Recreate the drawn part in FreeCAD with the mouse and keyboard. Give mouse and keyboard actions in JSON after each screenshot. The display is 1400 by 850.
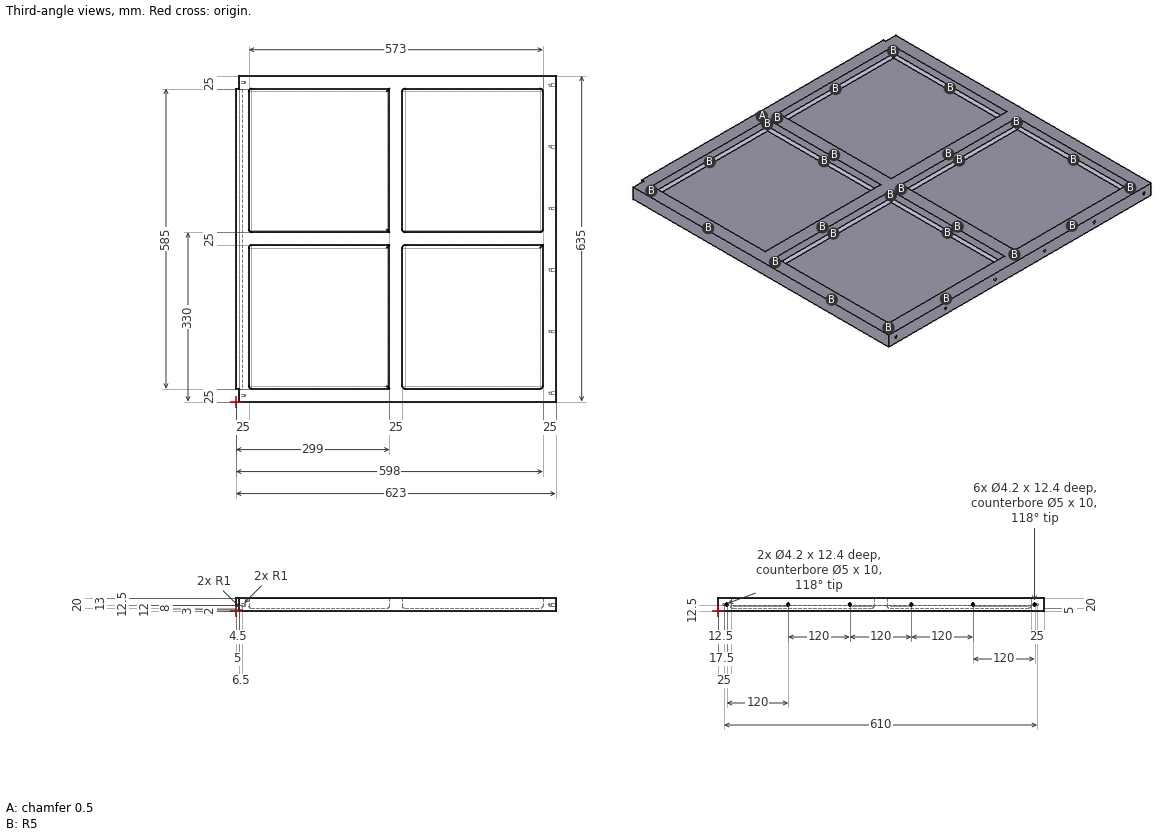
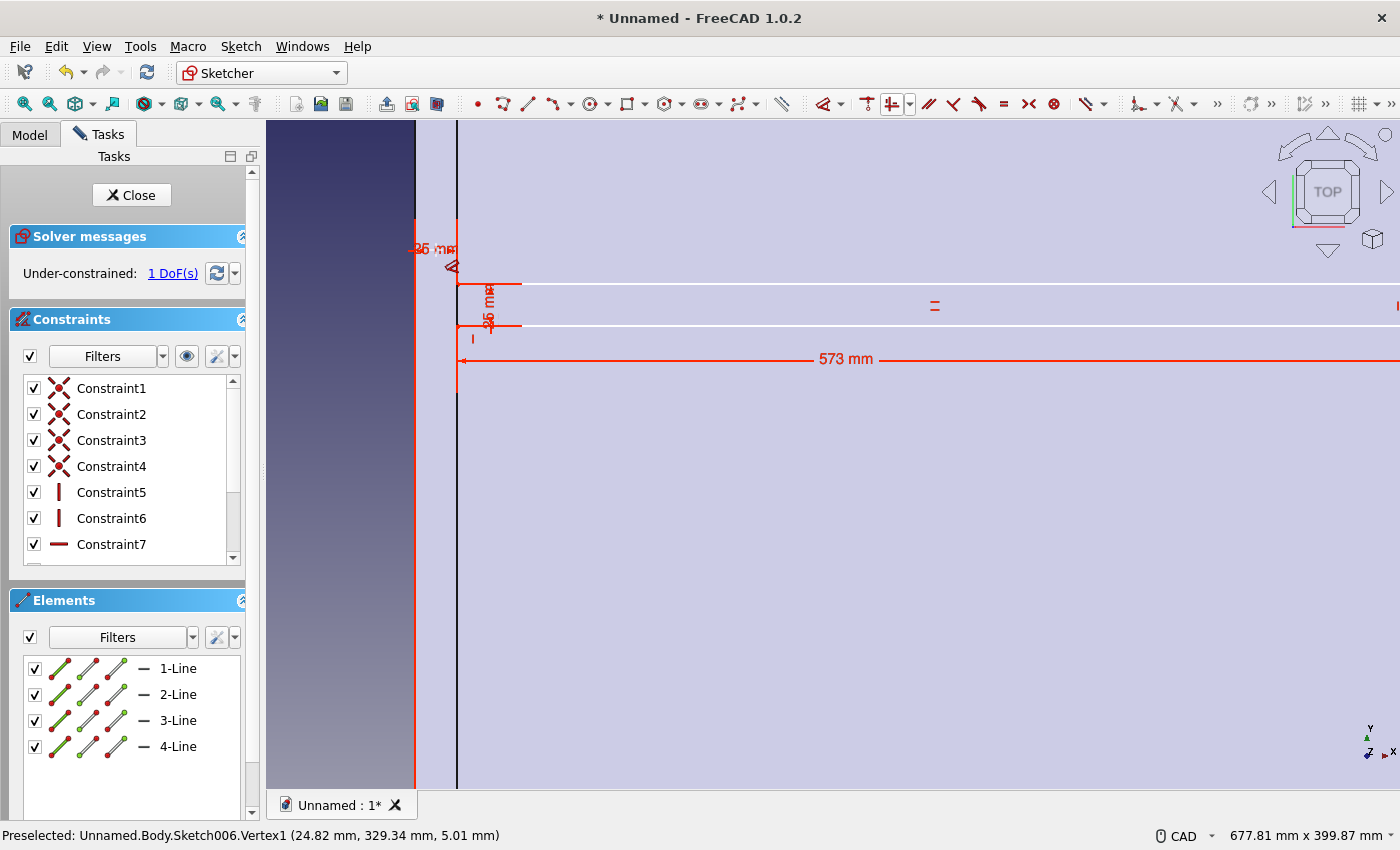
{"action": "left_click", "coordinate": [457, 284]}
{"action": "left_click", "coordinate": [381, 523]}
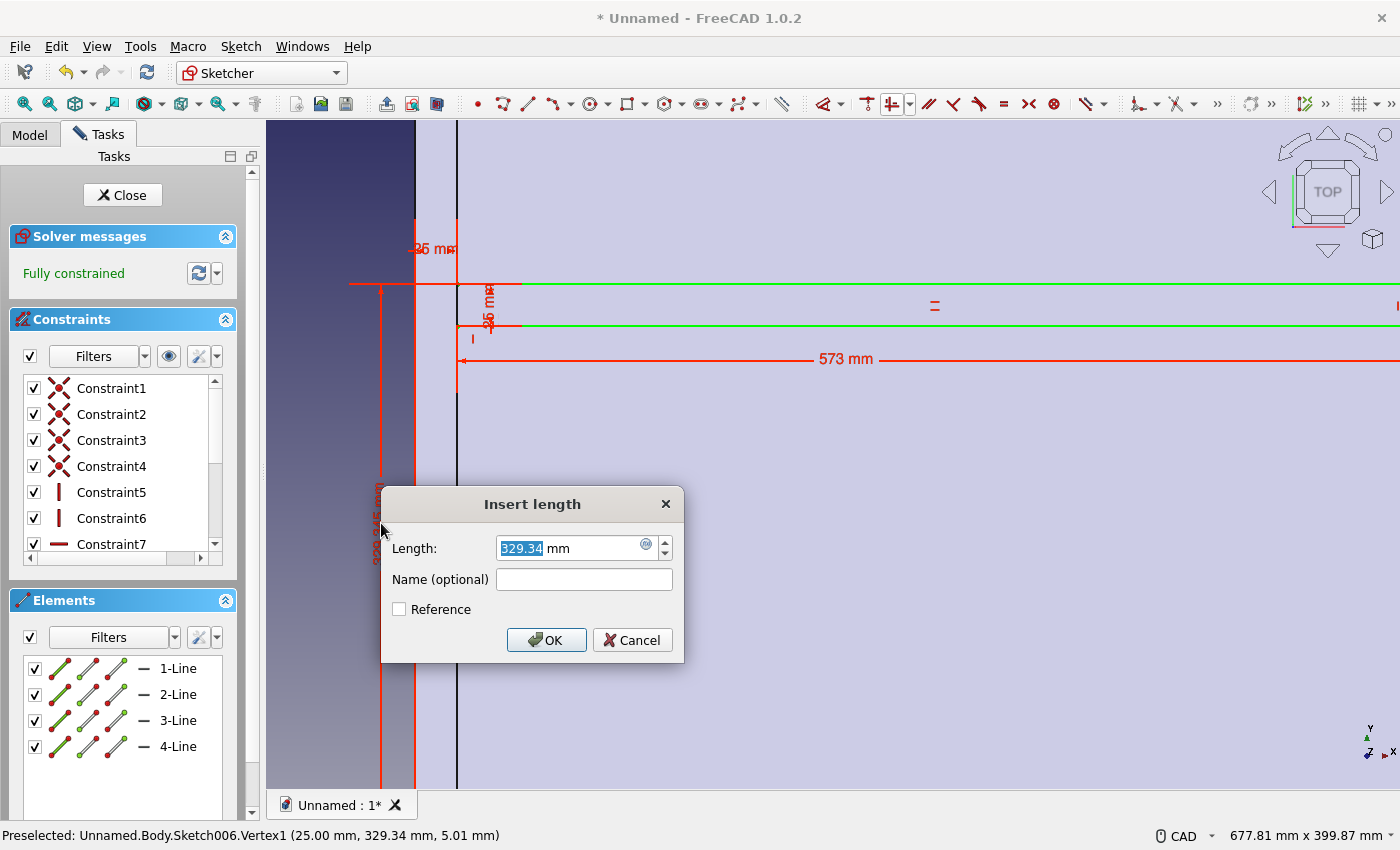
{"action": "type", "text": "330"}
{"action": "key", "text": "Return"}
{"action": "key", "text": "Escape"}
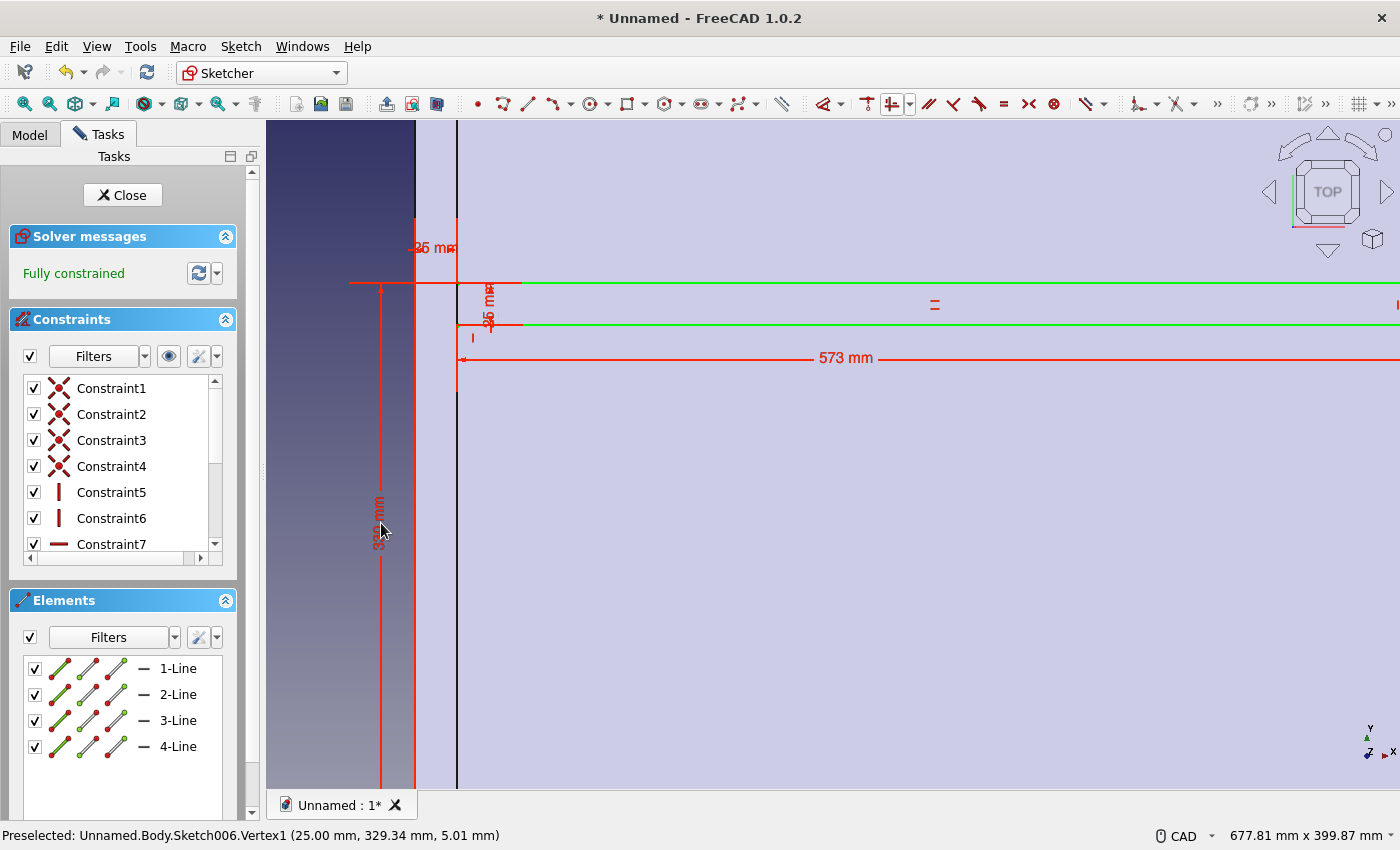
{"action": "left_click", "coordinate": [123, 195]}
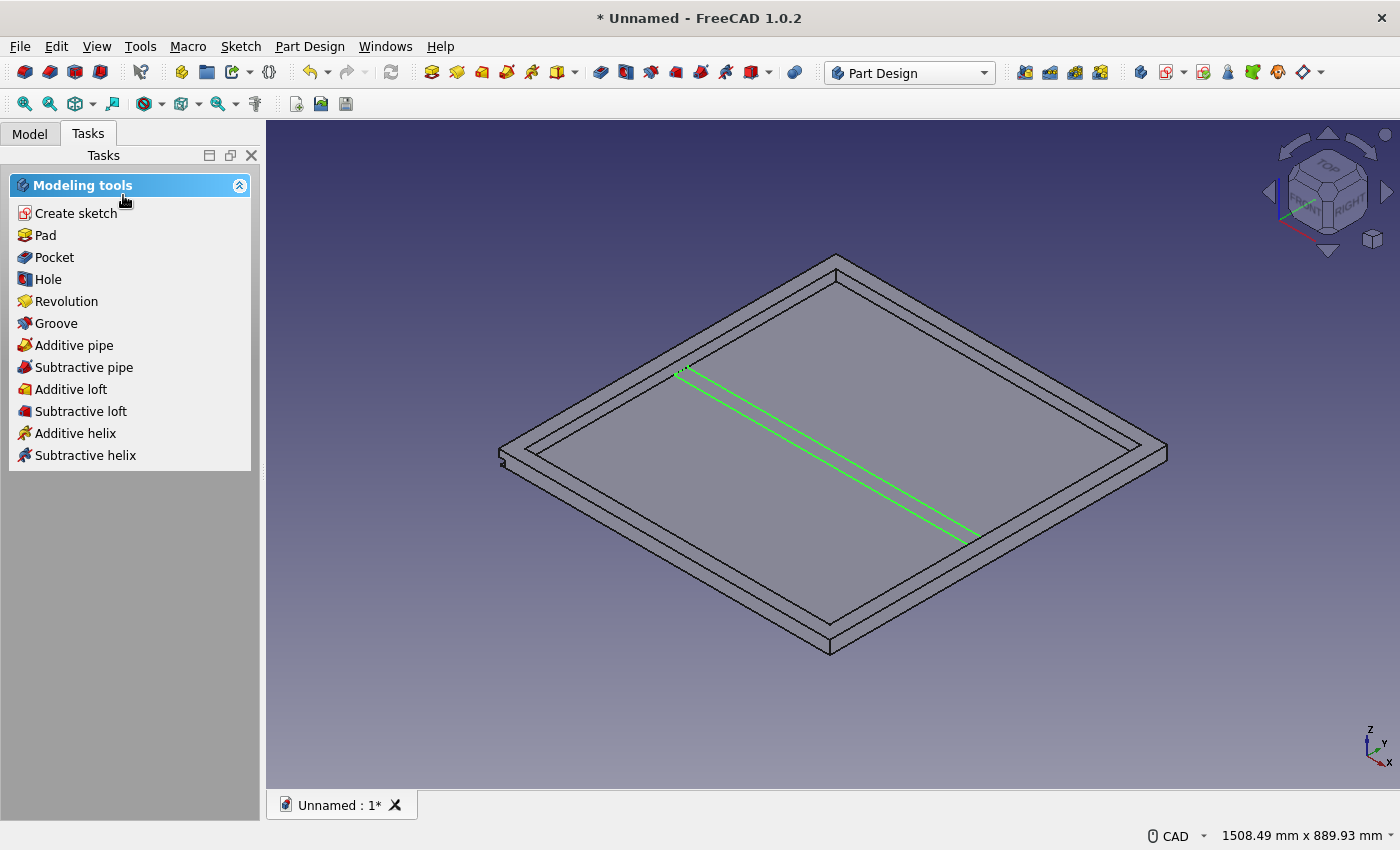
{"action": "left_click", "coordinate": [432, 72]}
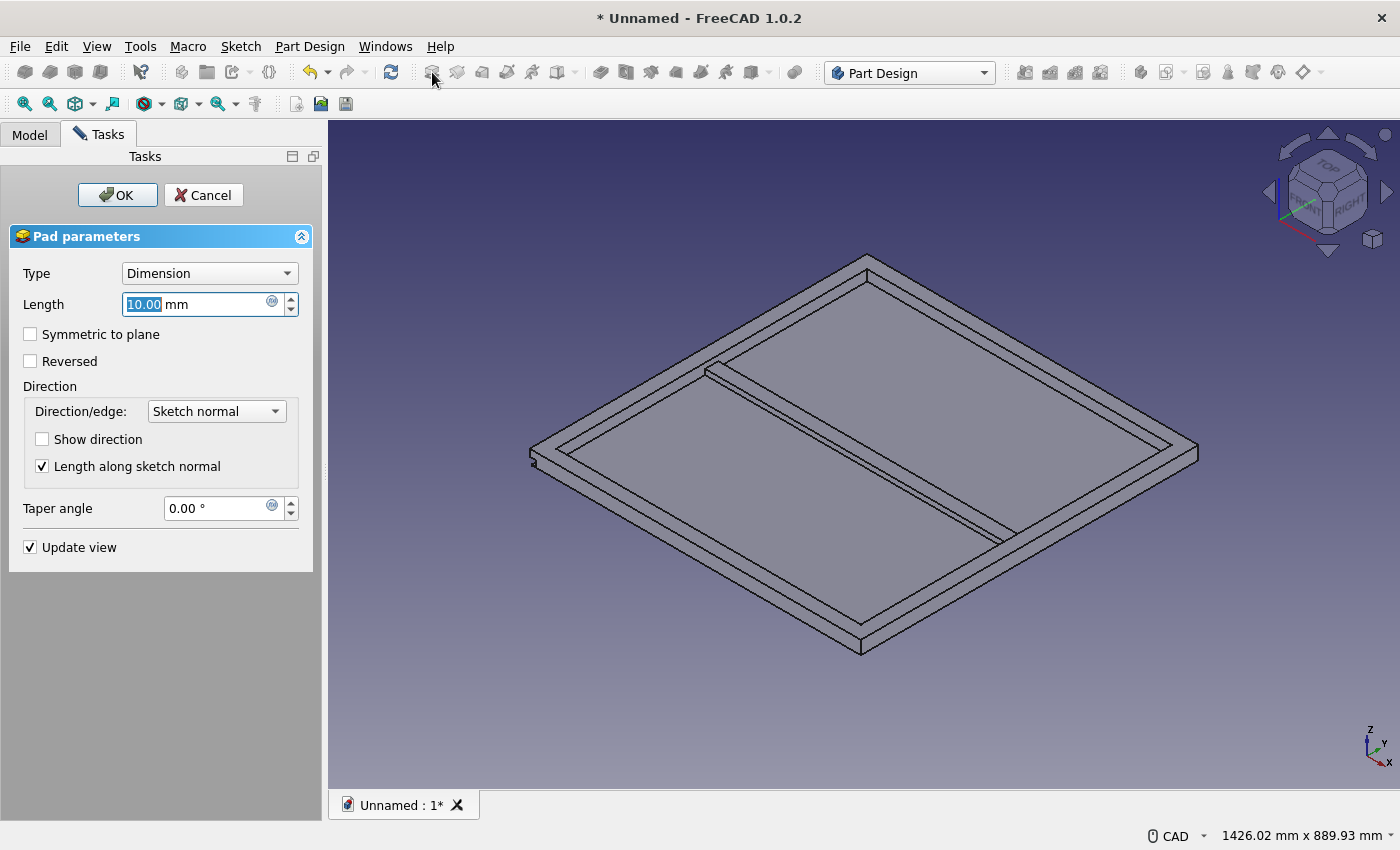
{"action": "type", "text": "20"}
{"action": "key", "text": "Tab"}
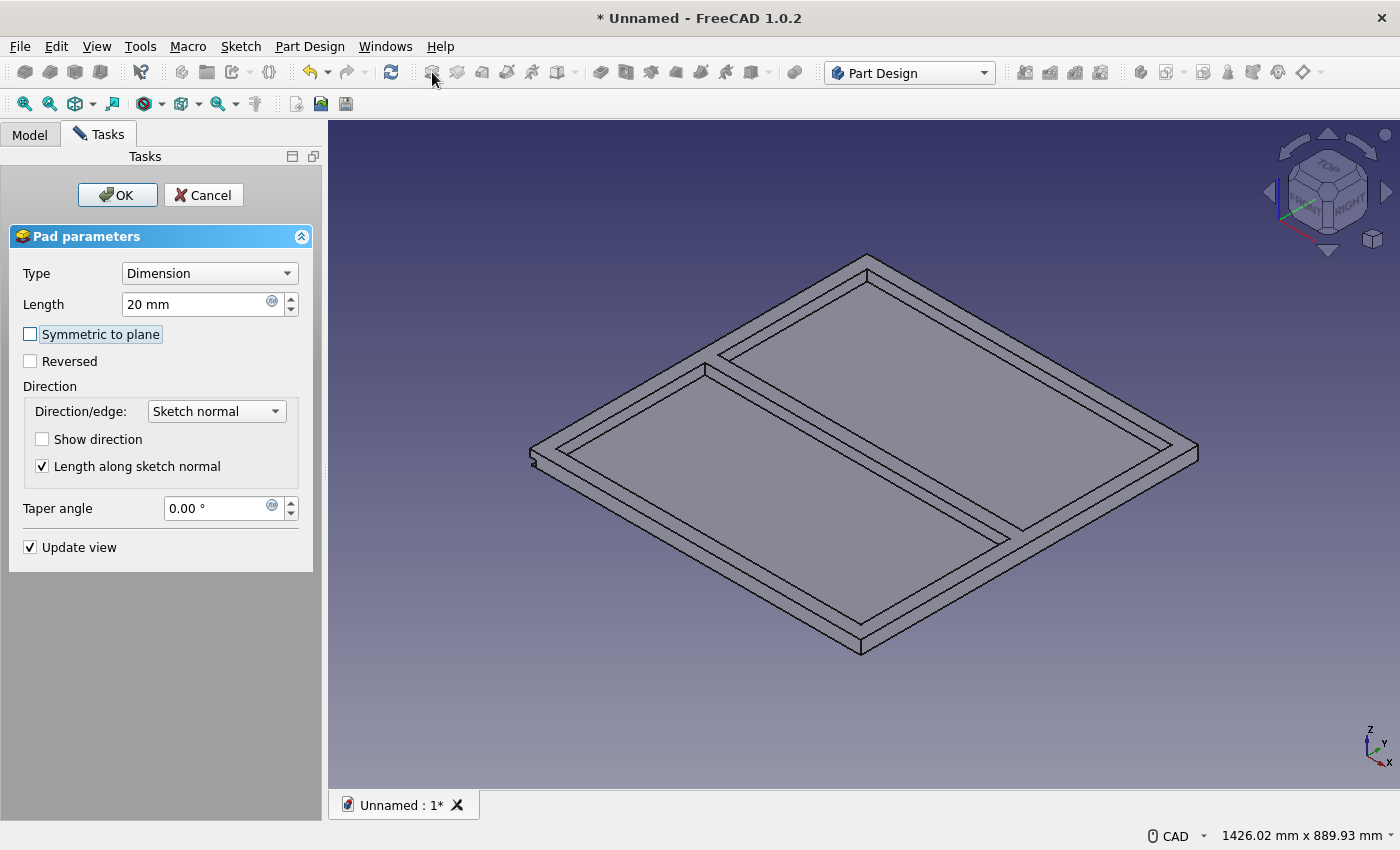
{"action": "left_click", "coordinate": [118, 195]}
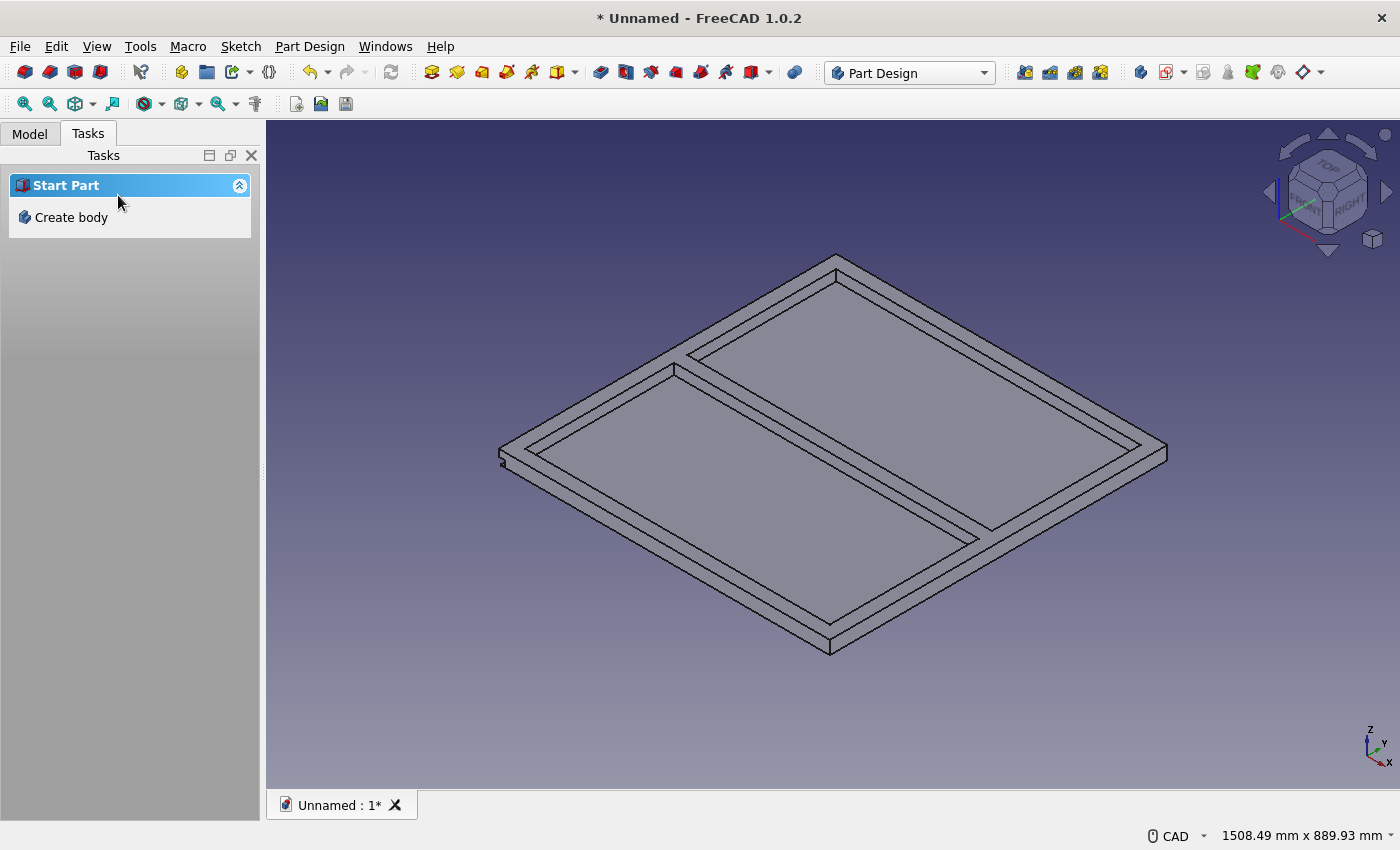
{"action": "left_click", "coordinate": [958, 436]}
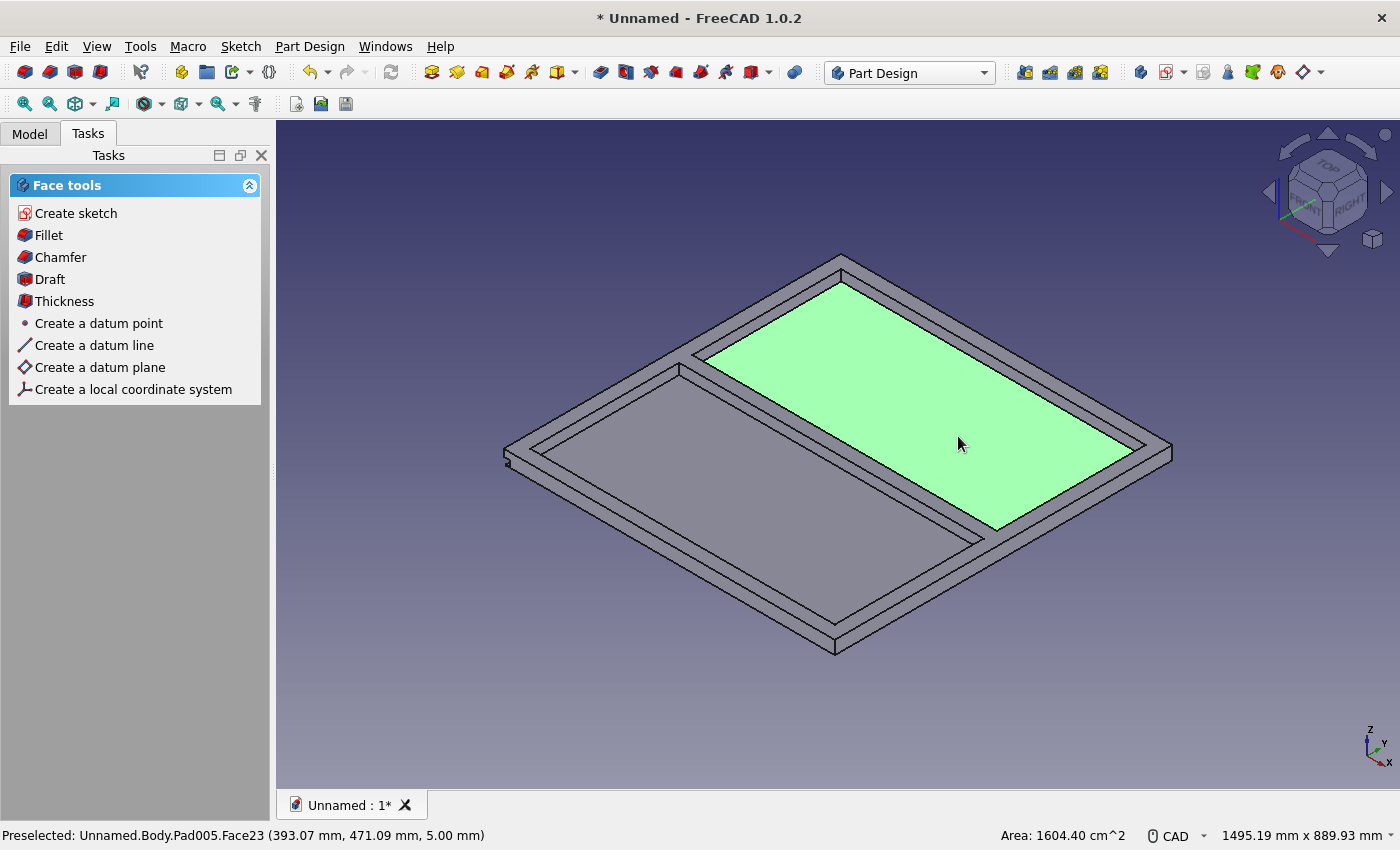
{"action": "left_click", "coordinate": [1166, 72]}